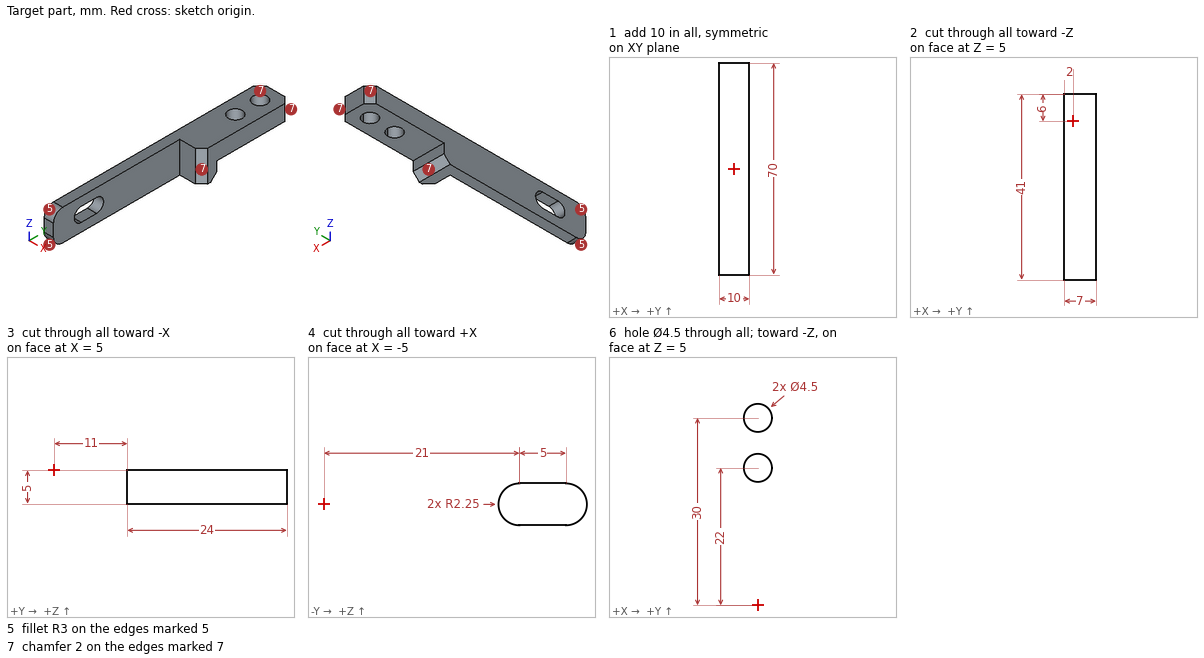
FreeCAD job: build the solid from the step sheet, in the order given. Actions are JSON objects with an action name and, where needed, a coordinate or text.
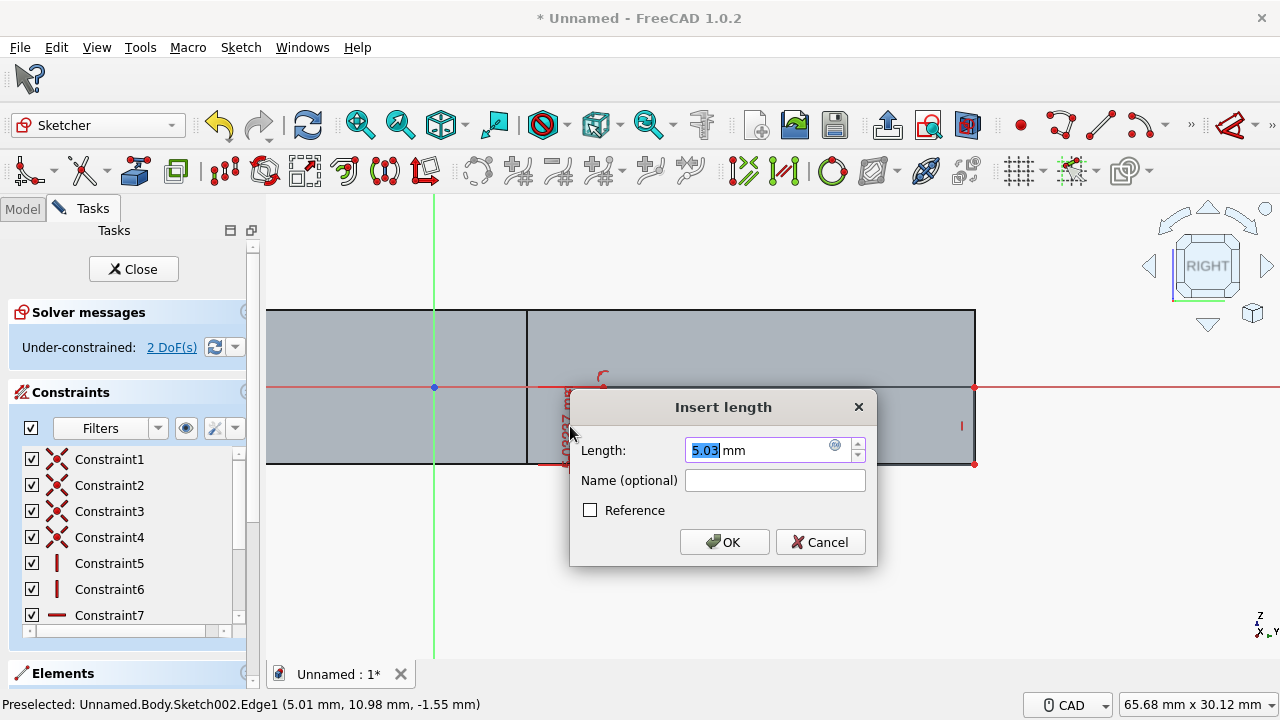
{"action": "type", "text": "5"}
{"action": "key", "text": "Return"}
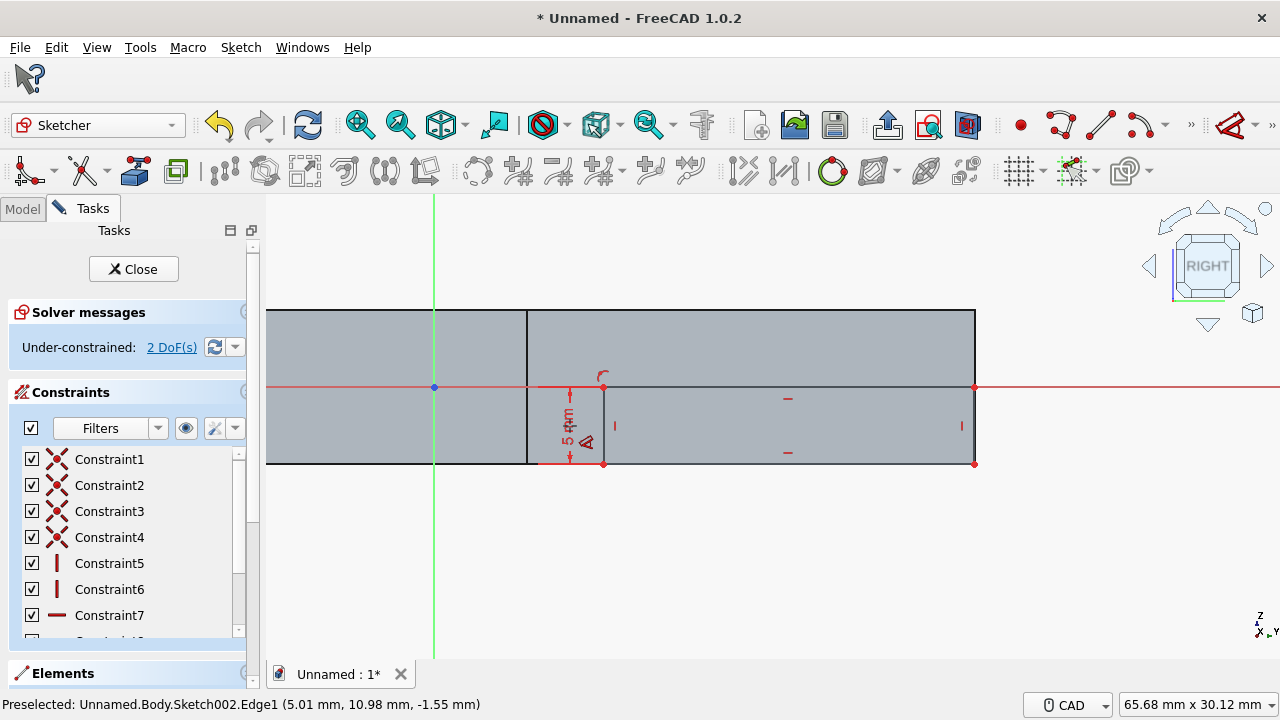
{"action": "left_click", "coordinate": [715, 464]}
{"action": "left_click", "coordinate": [789, 498]}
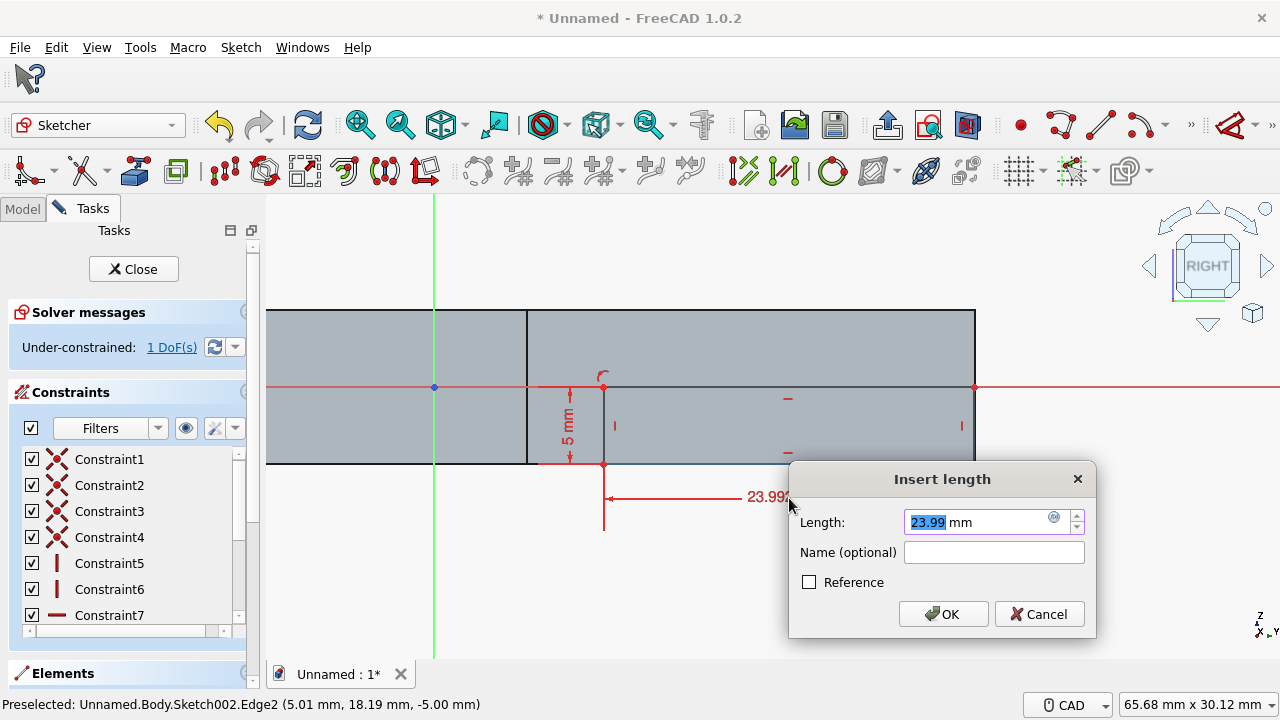
{"action": "type", "text": "24"}
{"action": "key", "text": "Return"}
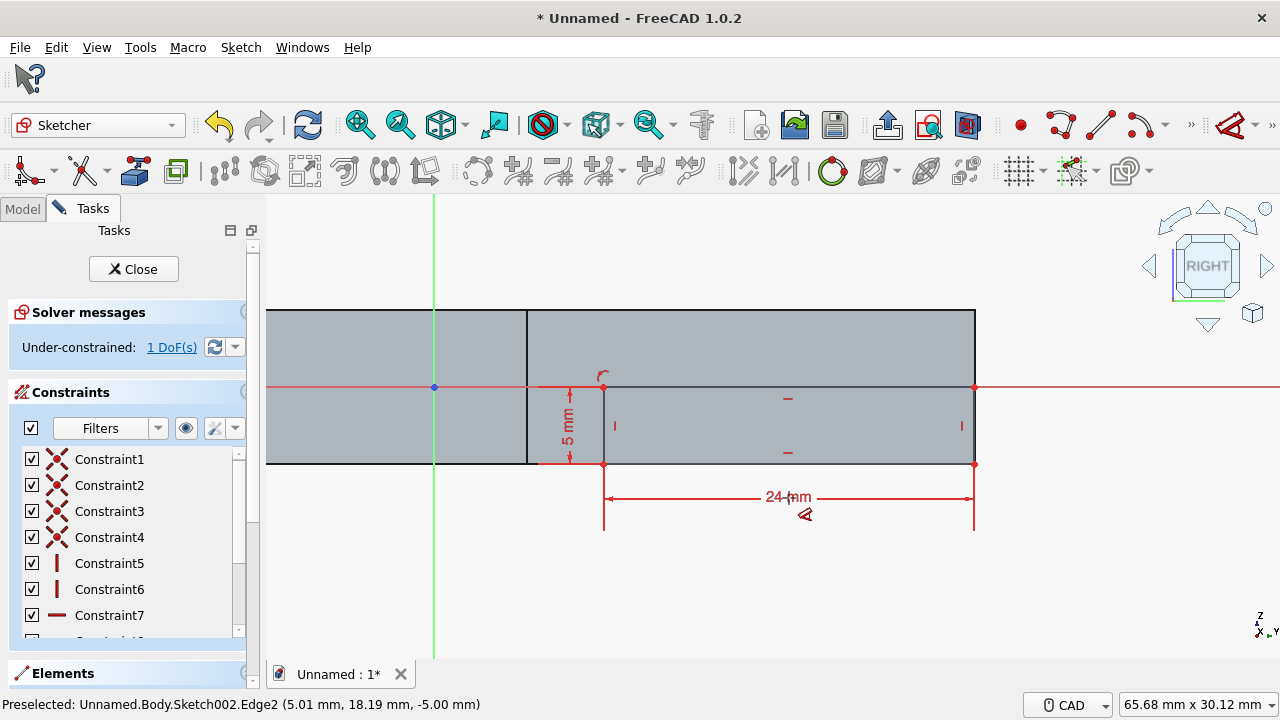
{"action": "left_click", "coordinate": [604, 387]}
{"action": "left_click", "coordinate": [519, 353]}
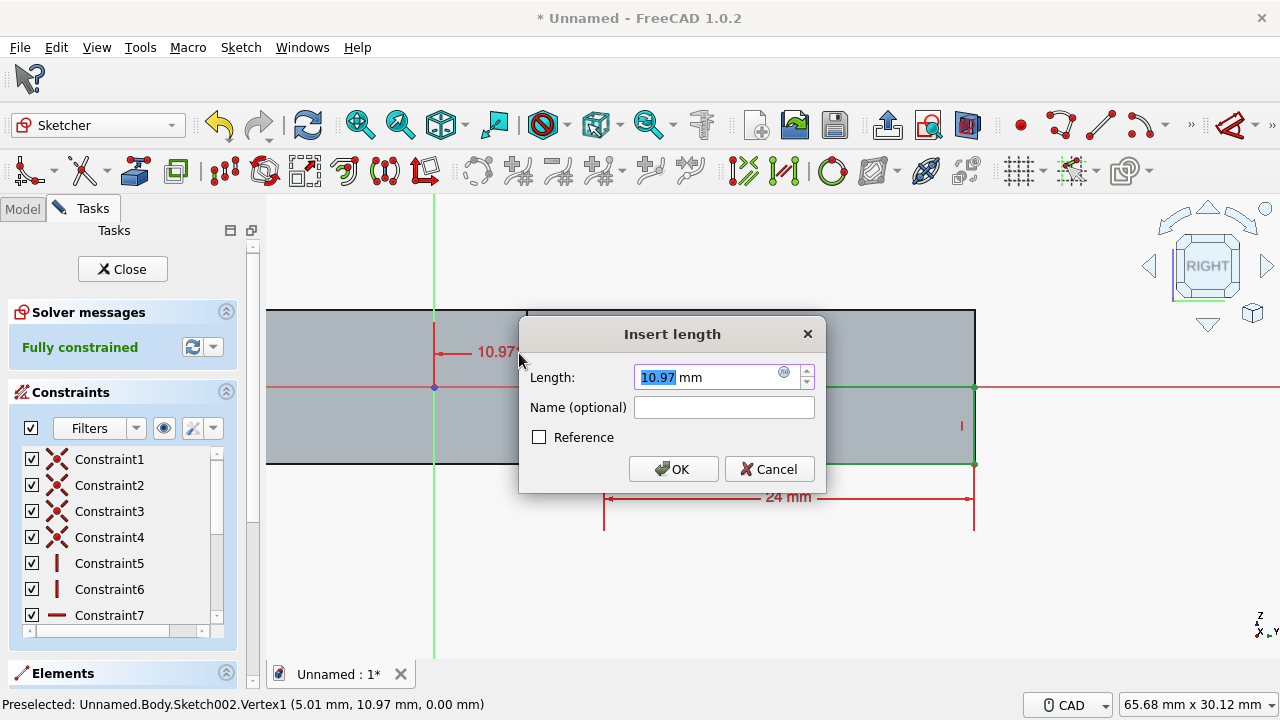
{"action": "type", "text": "11"}
{"action": "key", "text": "Return"}
{"action": "key", "text": "Escape"}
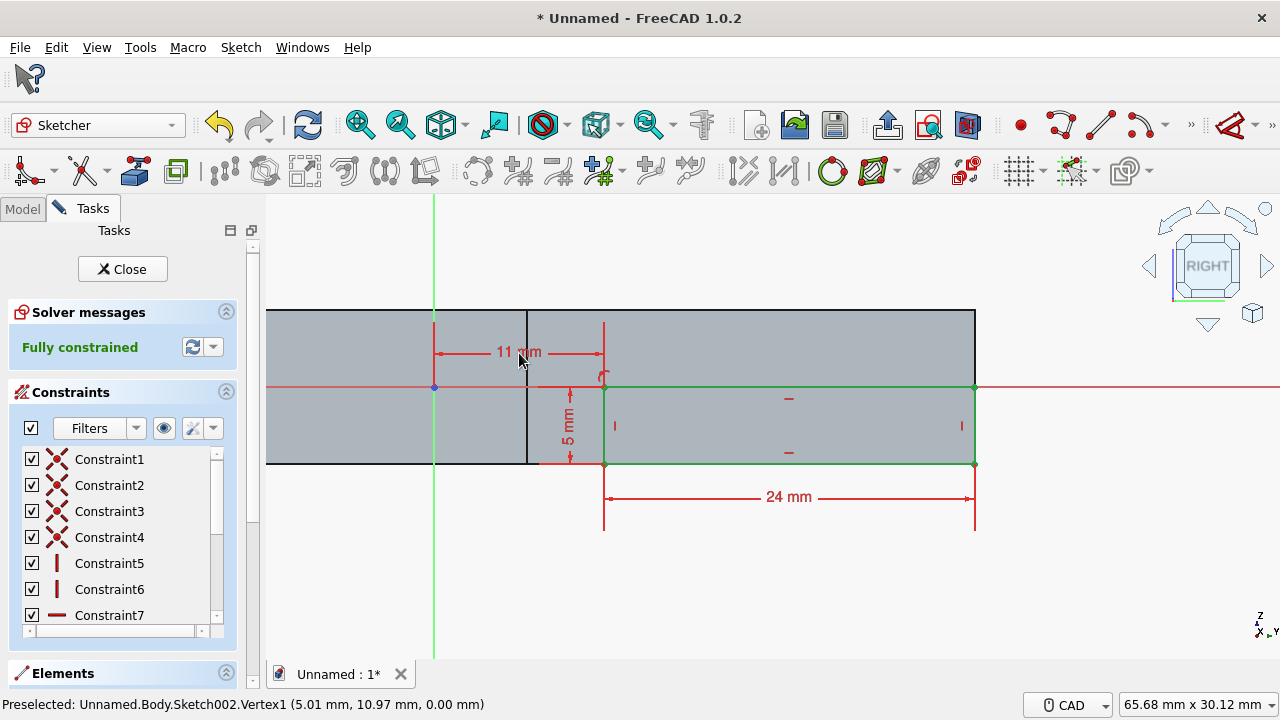
{"action": "left_click", "coordinate": [123, 269]}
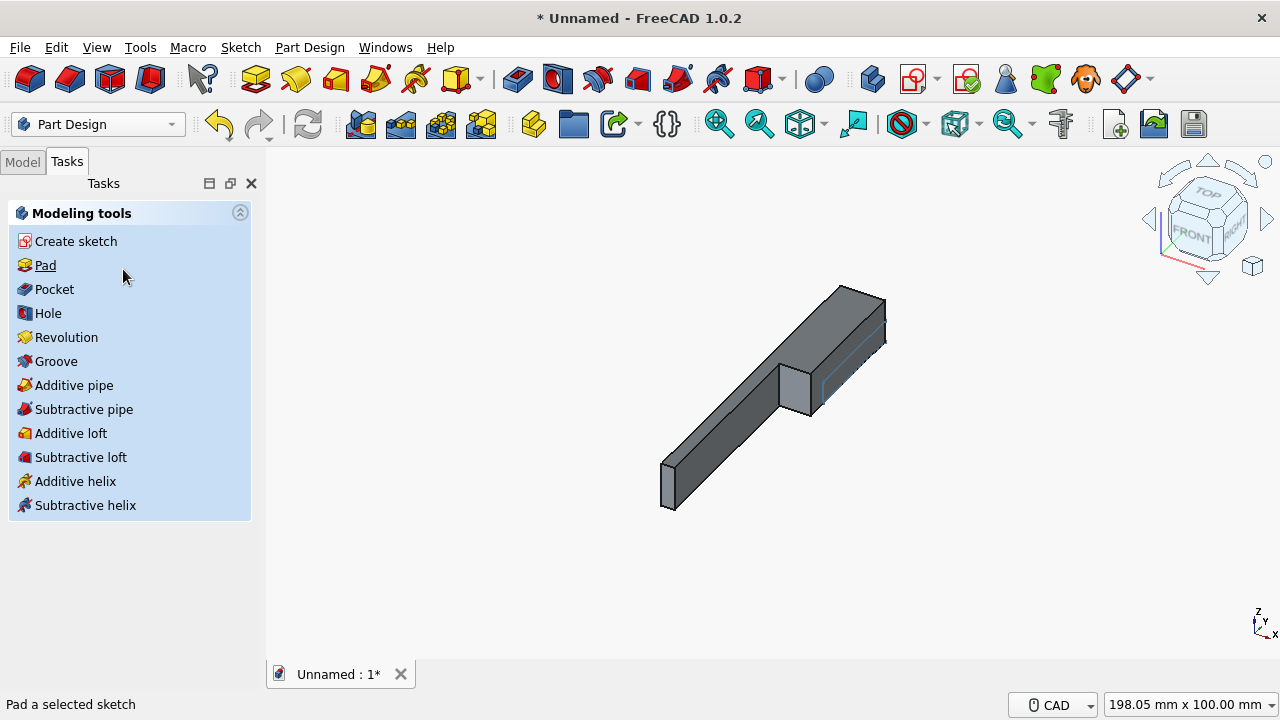
{"action": "left_click", "coordinate": [518, 80]}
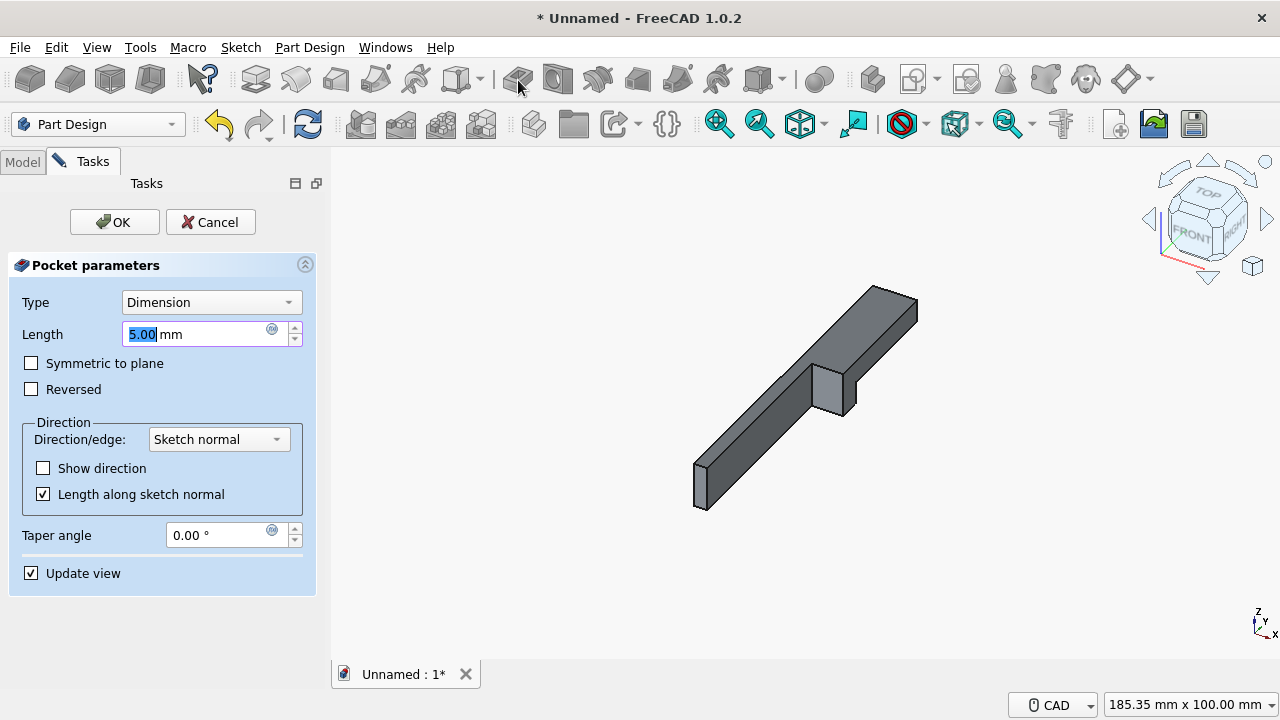
{"action": "left_click", "coordinate": [212, 302]}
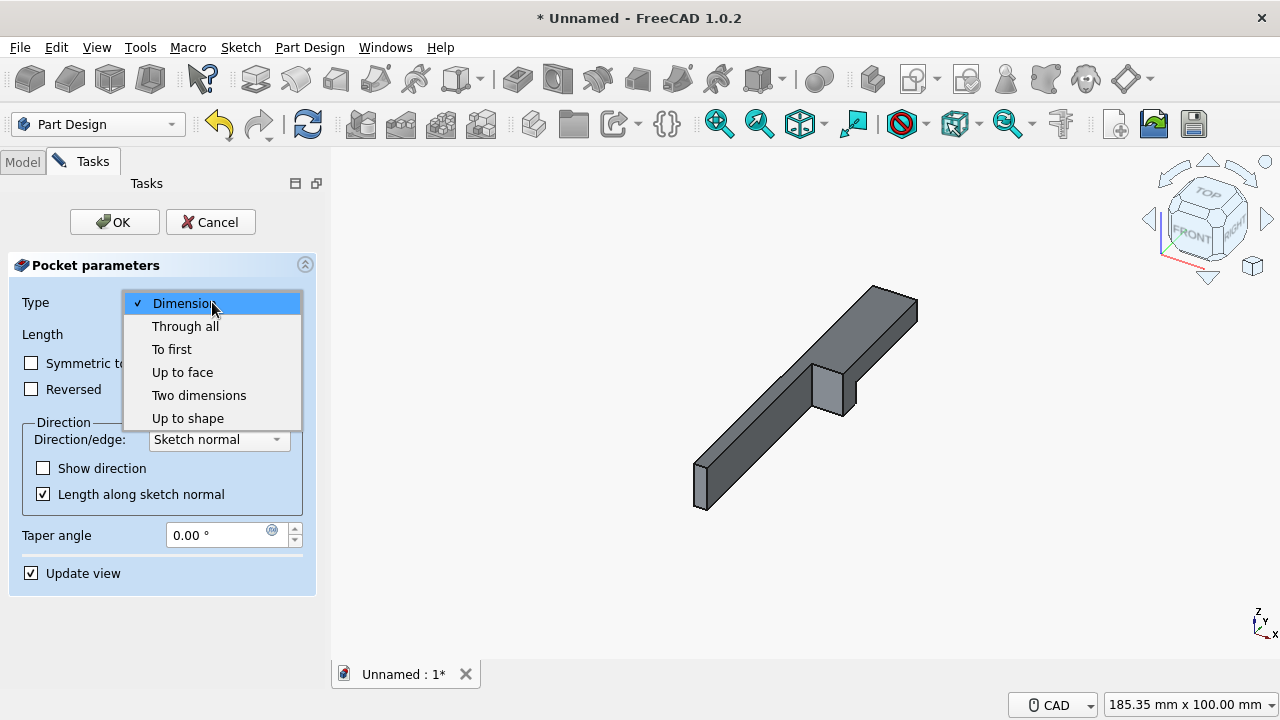
{"action": "left_click", "coordinate": [212, 326]}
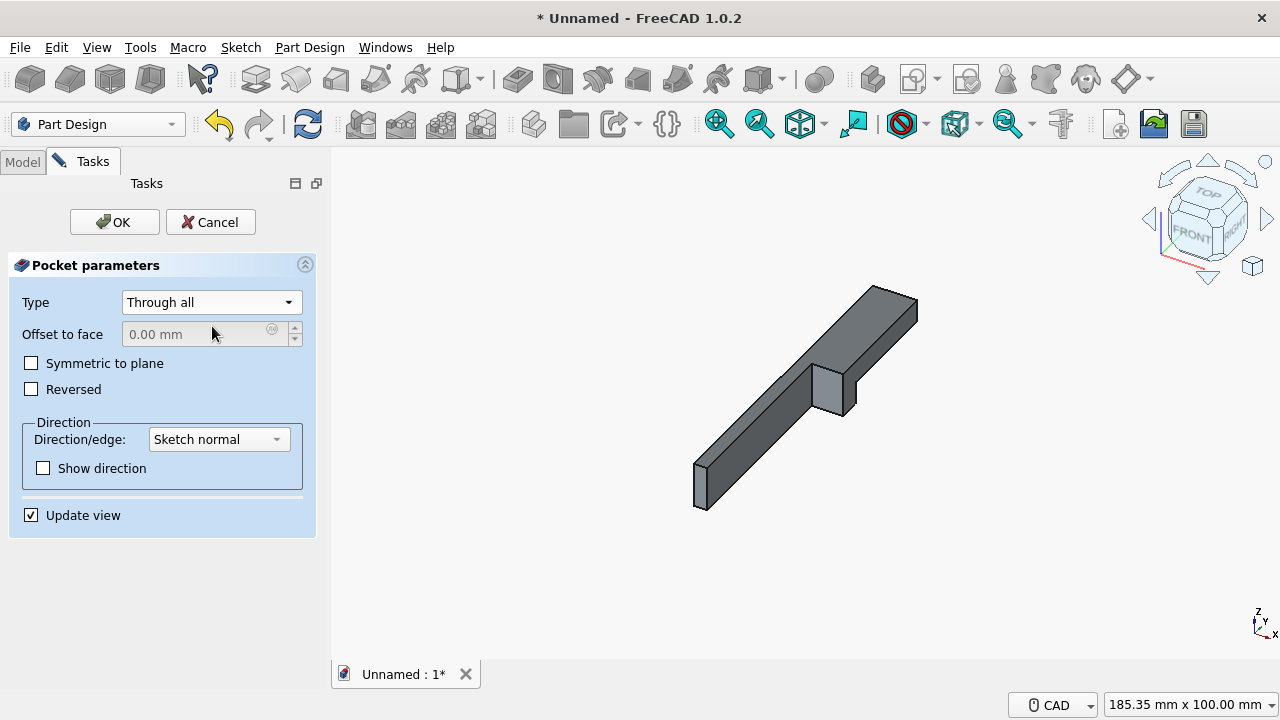
{"action": "left_click", "coordinate": [115, 222]}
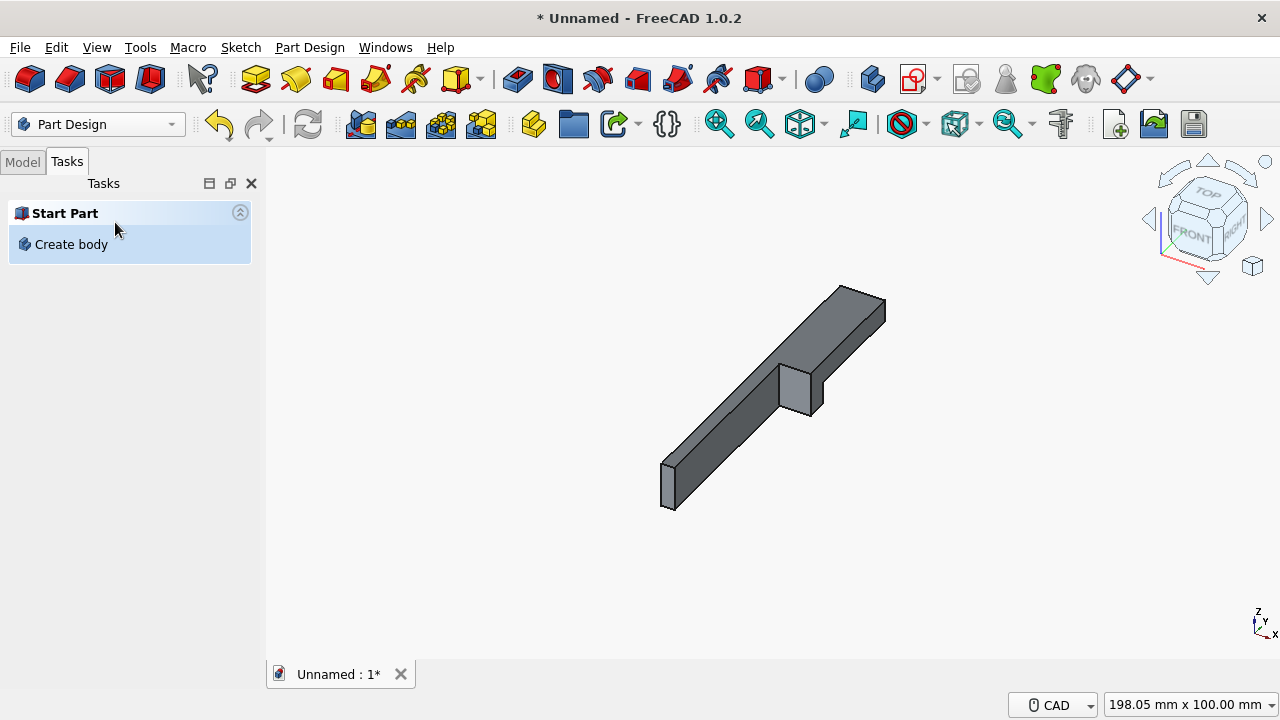
{"action": "key", "text": "6"}